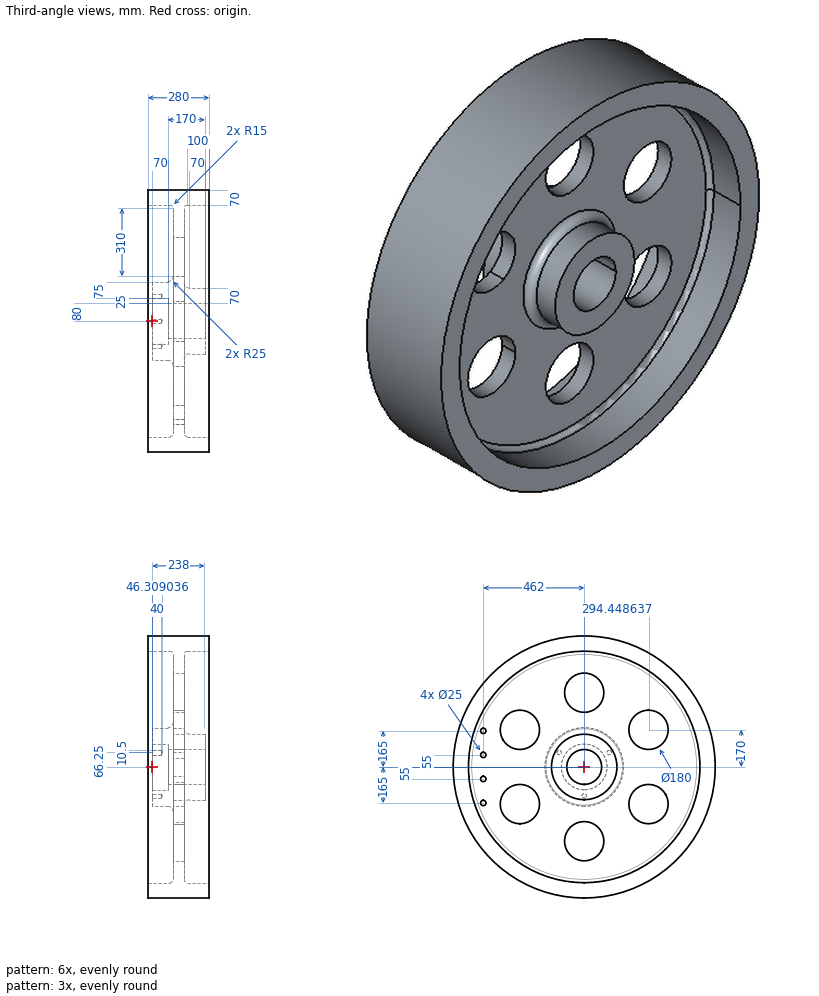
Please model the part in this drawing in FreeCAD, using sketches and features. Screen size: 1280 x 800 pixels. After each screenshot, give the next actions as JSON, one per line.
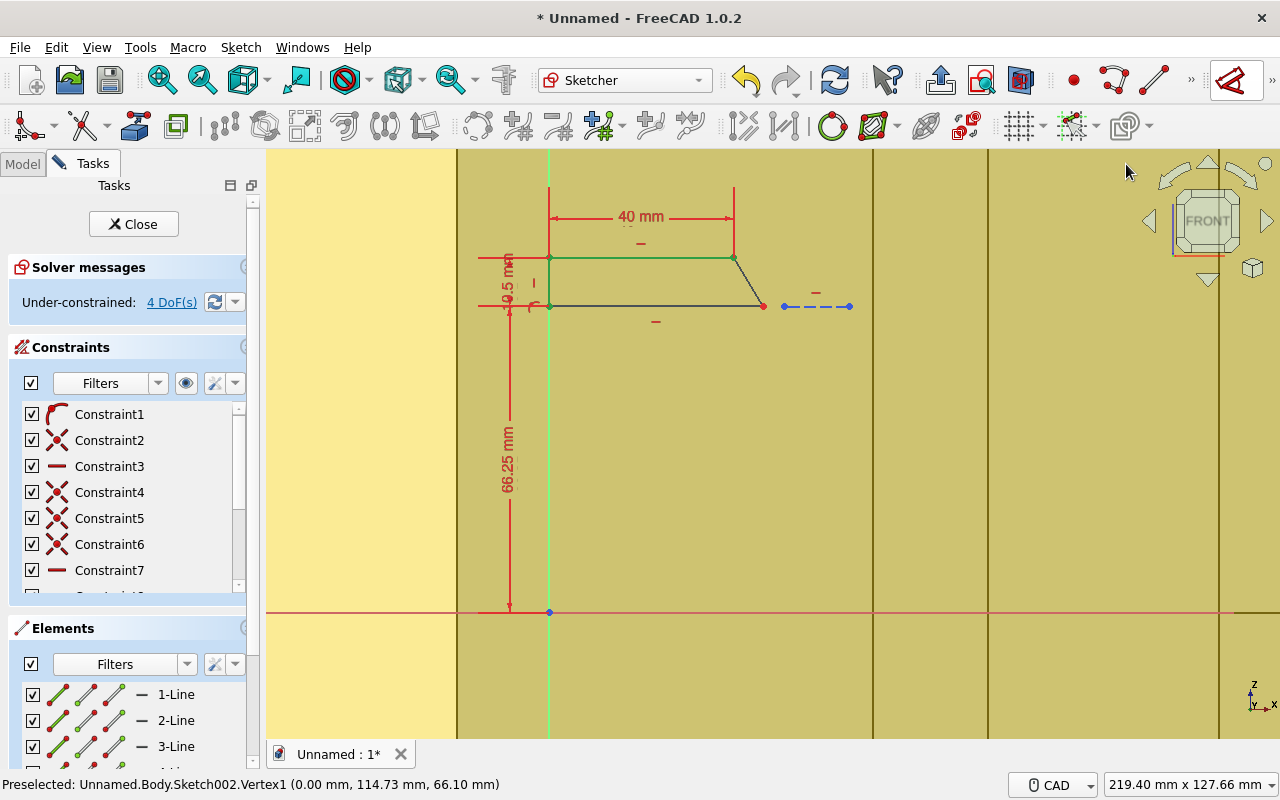
{"action": "left_click", "coordinate": [784, 307]}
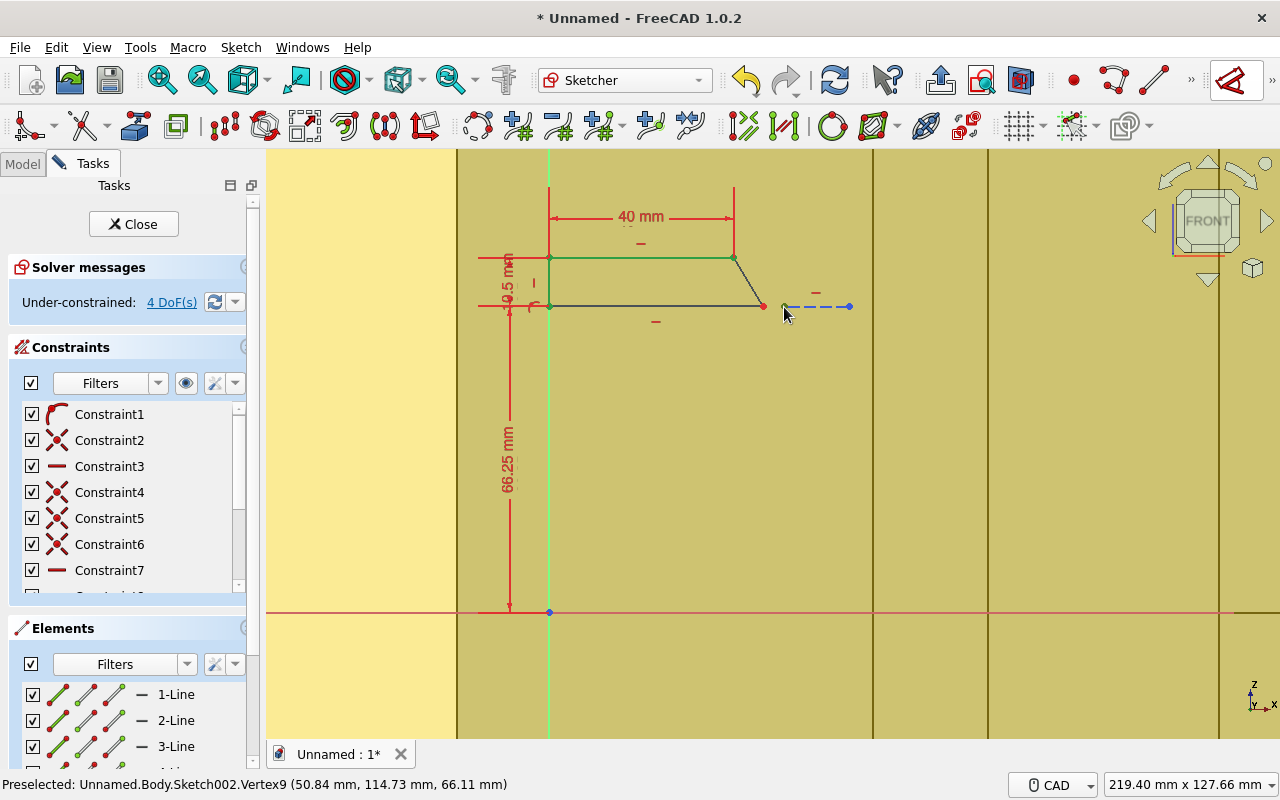
{"action": "key", "text": "i"}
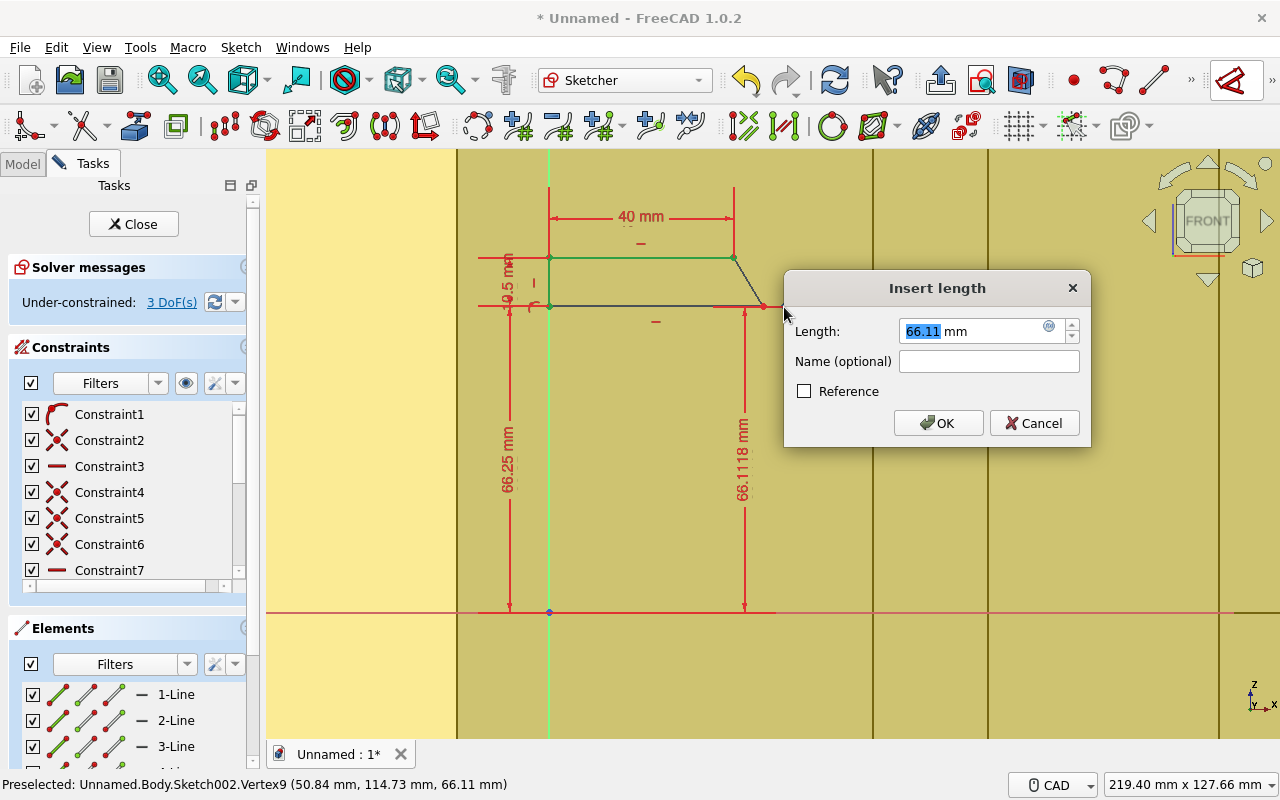
{"action": "type", "text": "66.25"}
{"action": "key", "text": "Return"}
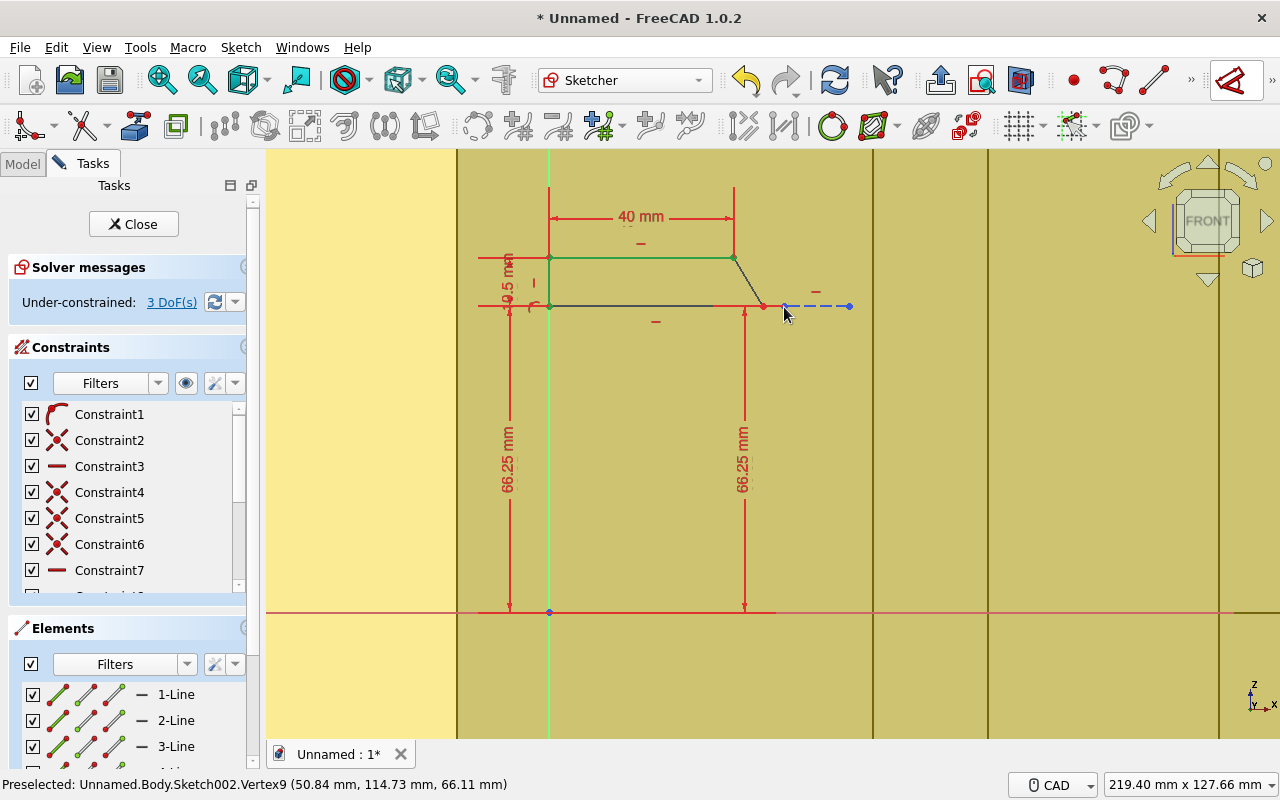
{"action": "left_click", "coordinate": [699, 306]}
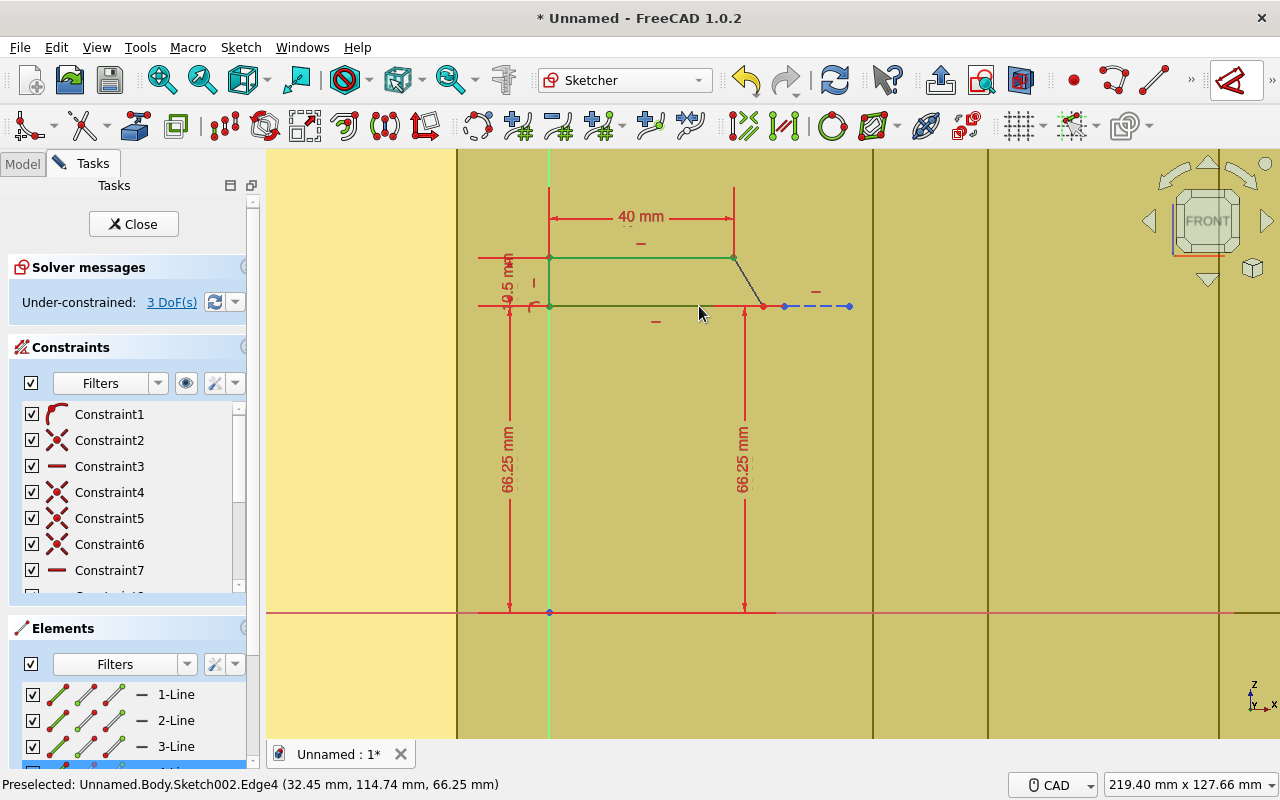
{"action": "left_click", "coordinate": [1258, 80]}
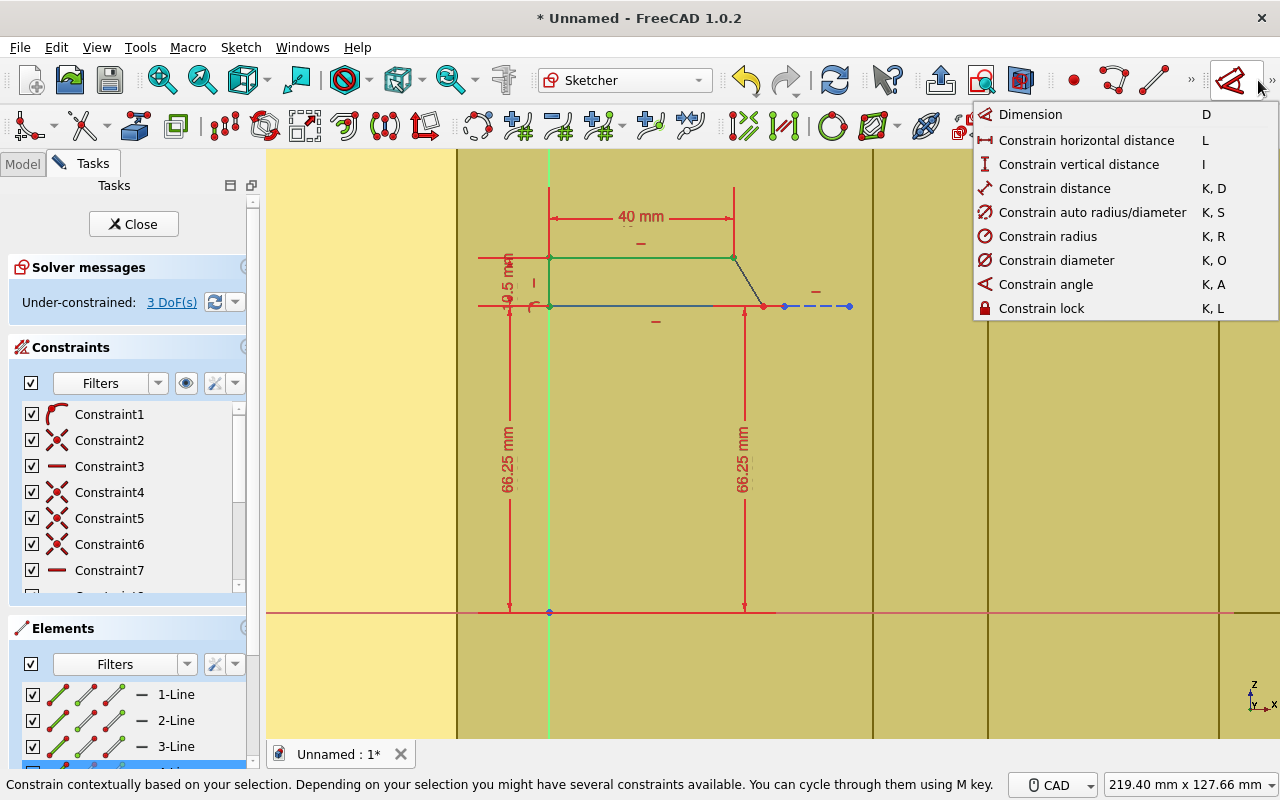
{"action": "left_click", "coordinate": [1126, 140]}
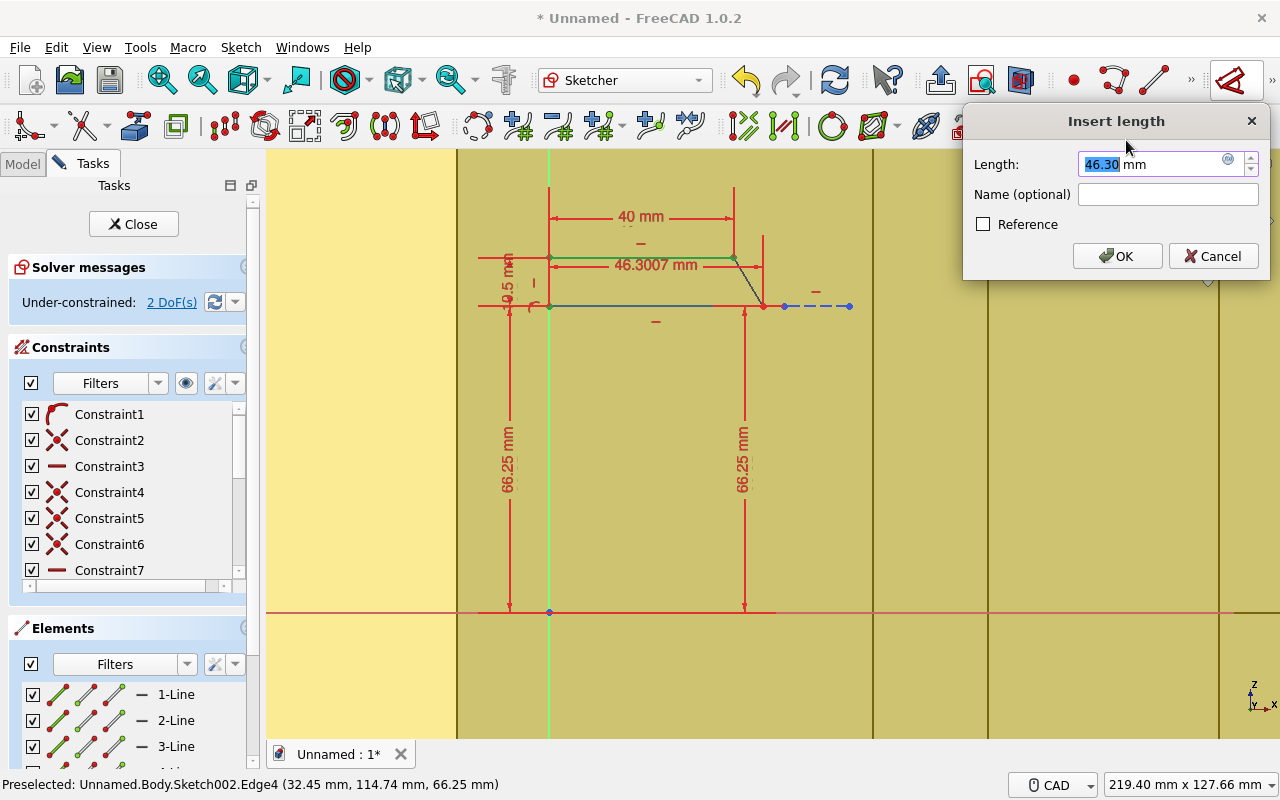
{"action": "type", "text": "46.309036"}
{"action": "key", "text": "Return"}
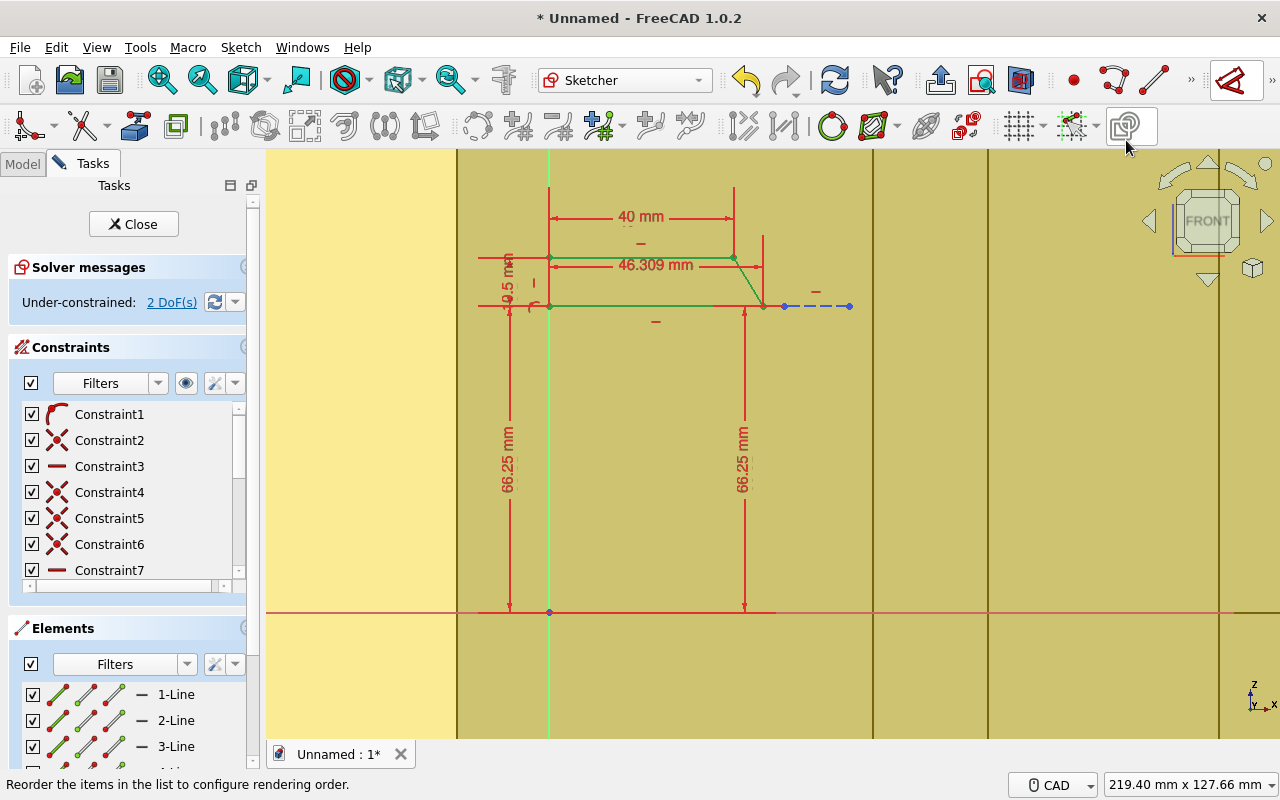
{"action": "left_click", "coordinate": [134, 224]}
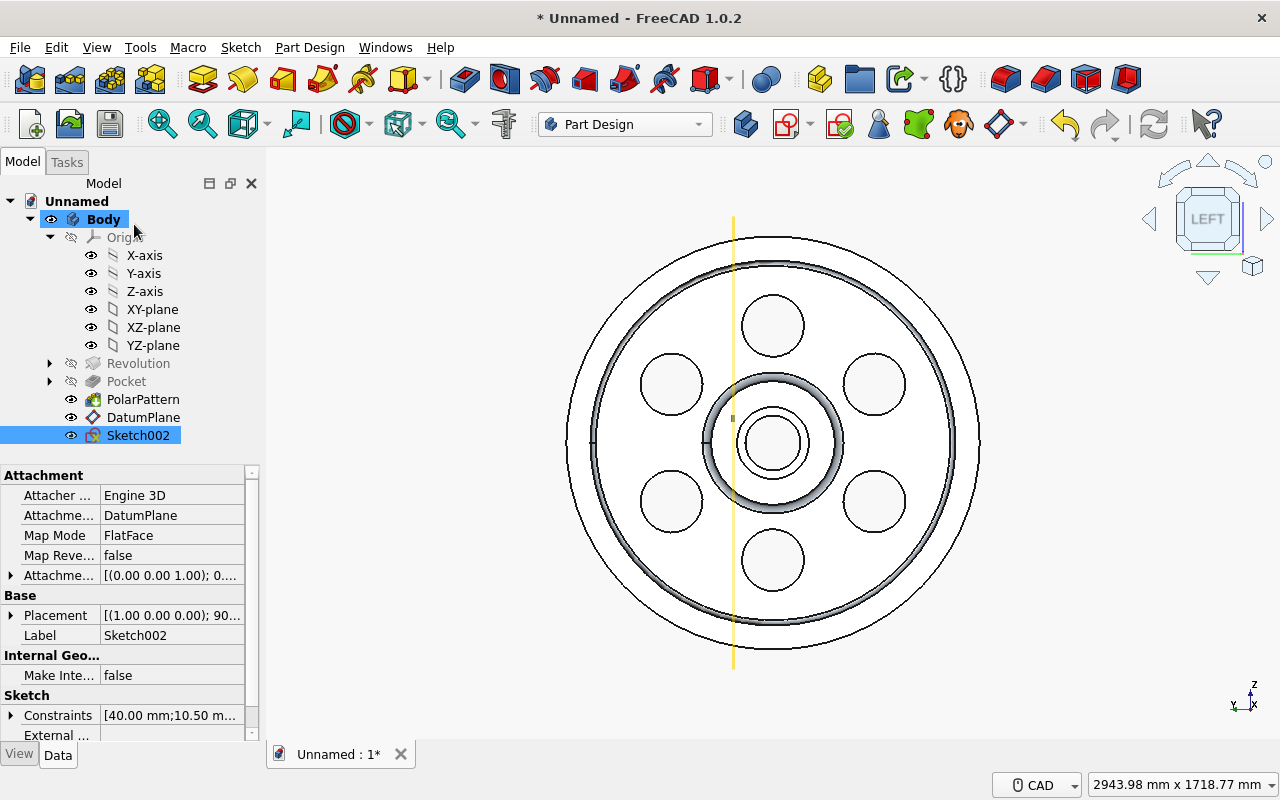
{"action": "left_click", "coordinate": [546, 80]}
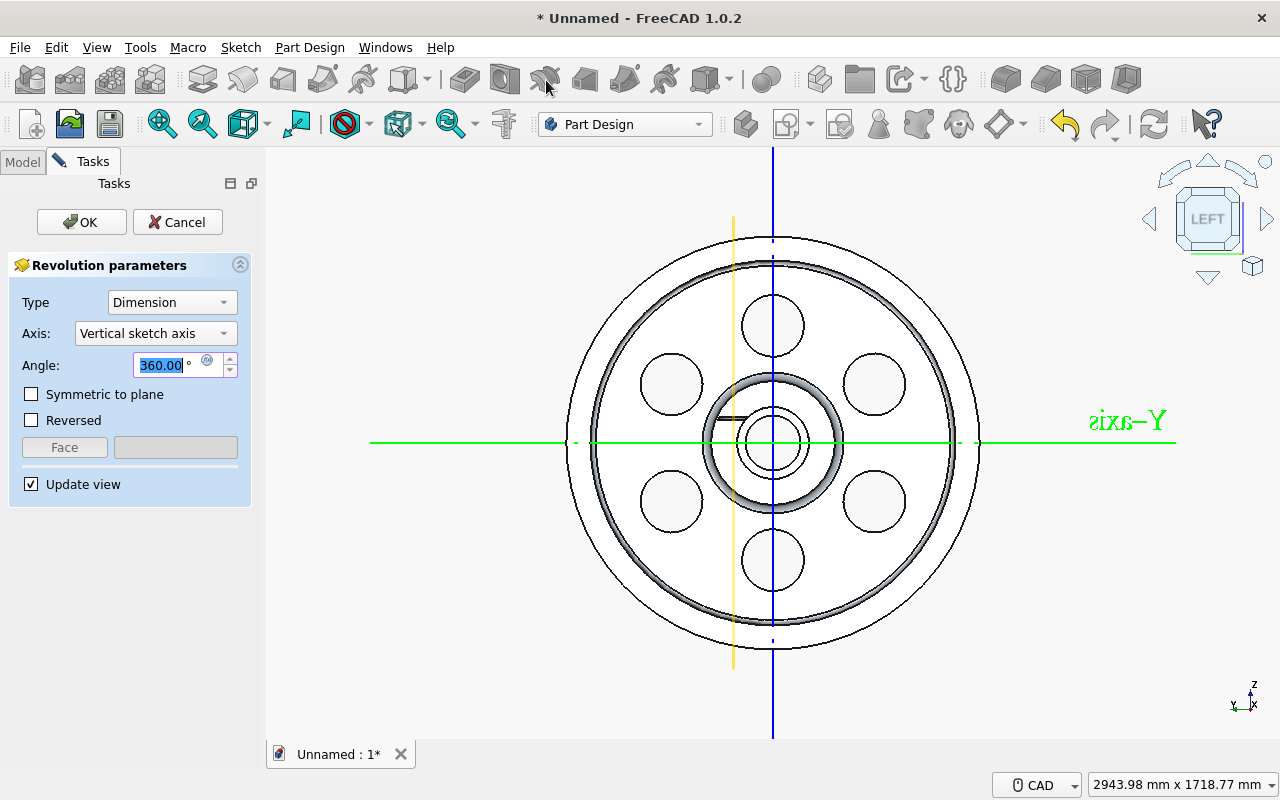
{"action": "left_click", "coordinate": [156, 334]}